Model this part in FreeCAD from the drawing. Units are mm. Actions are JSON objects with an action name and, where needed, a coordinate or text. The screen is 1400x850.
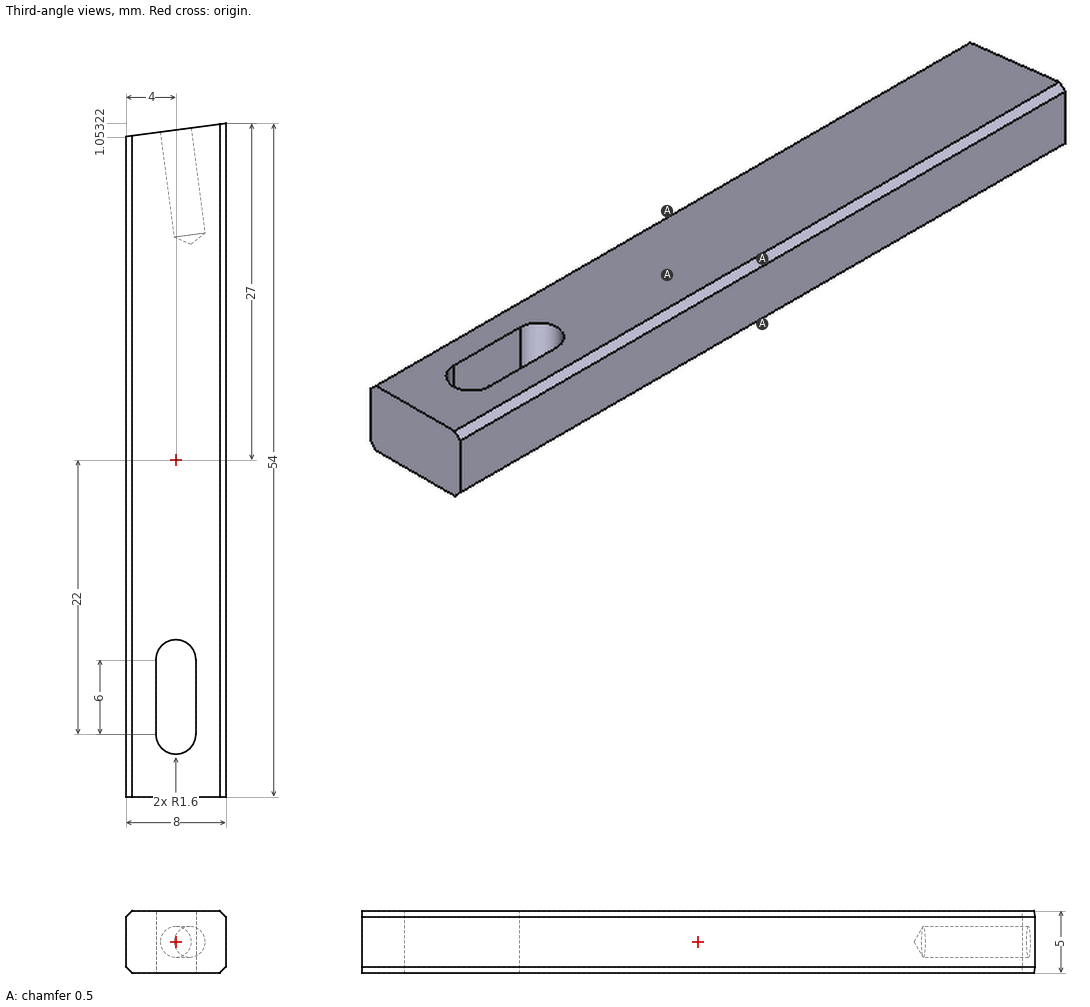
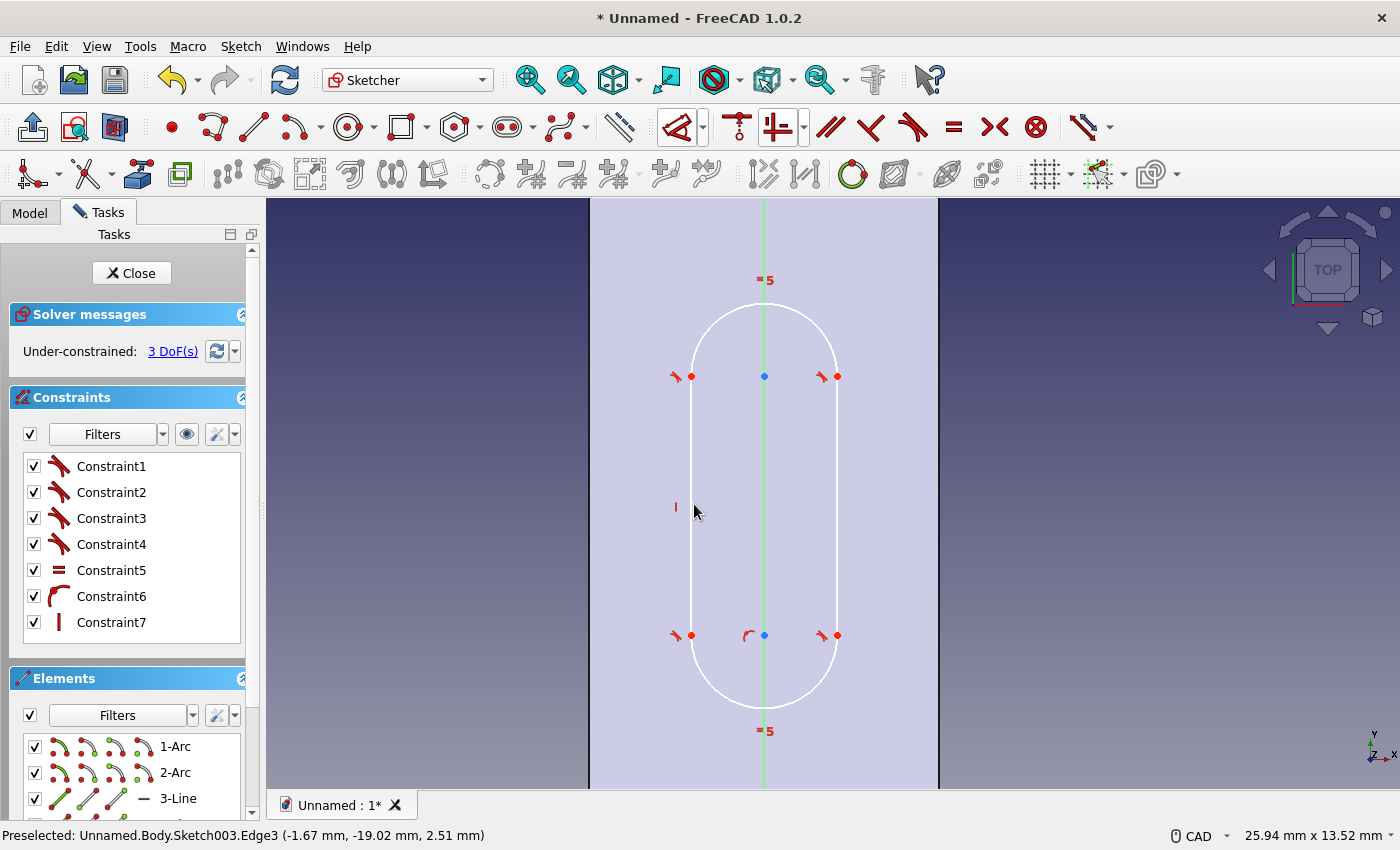
{"action": "left_click", "coordinate": [721, 694]}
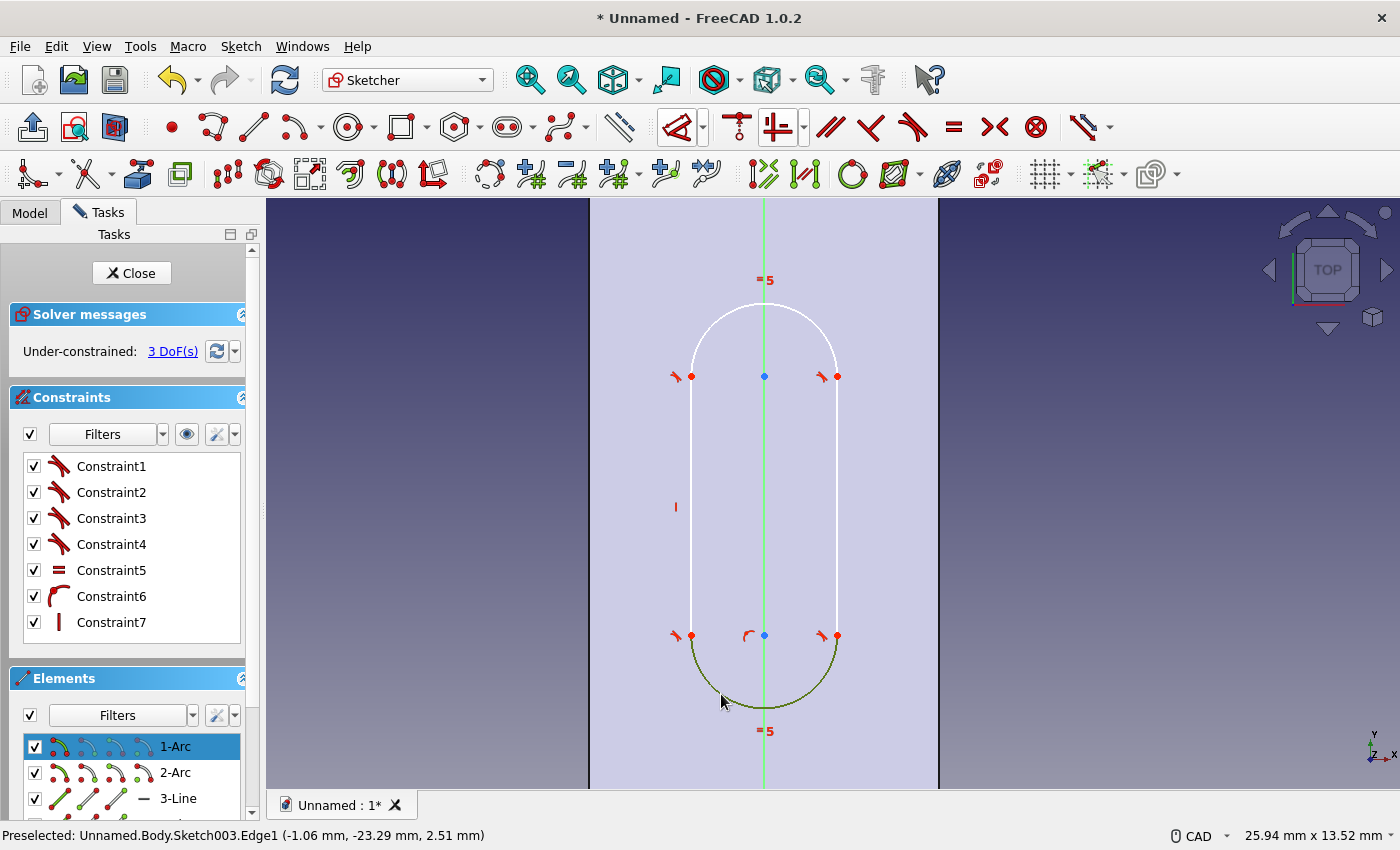
{"action": "key", "text": "k r"}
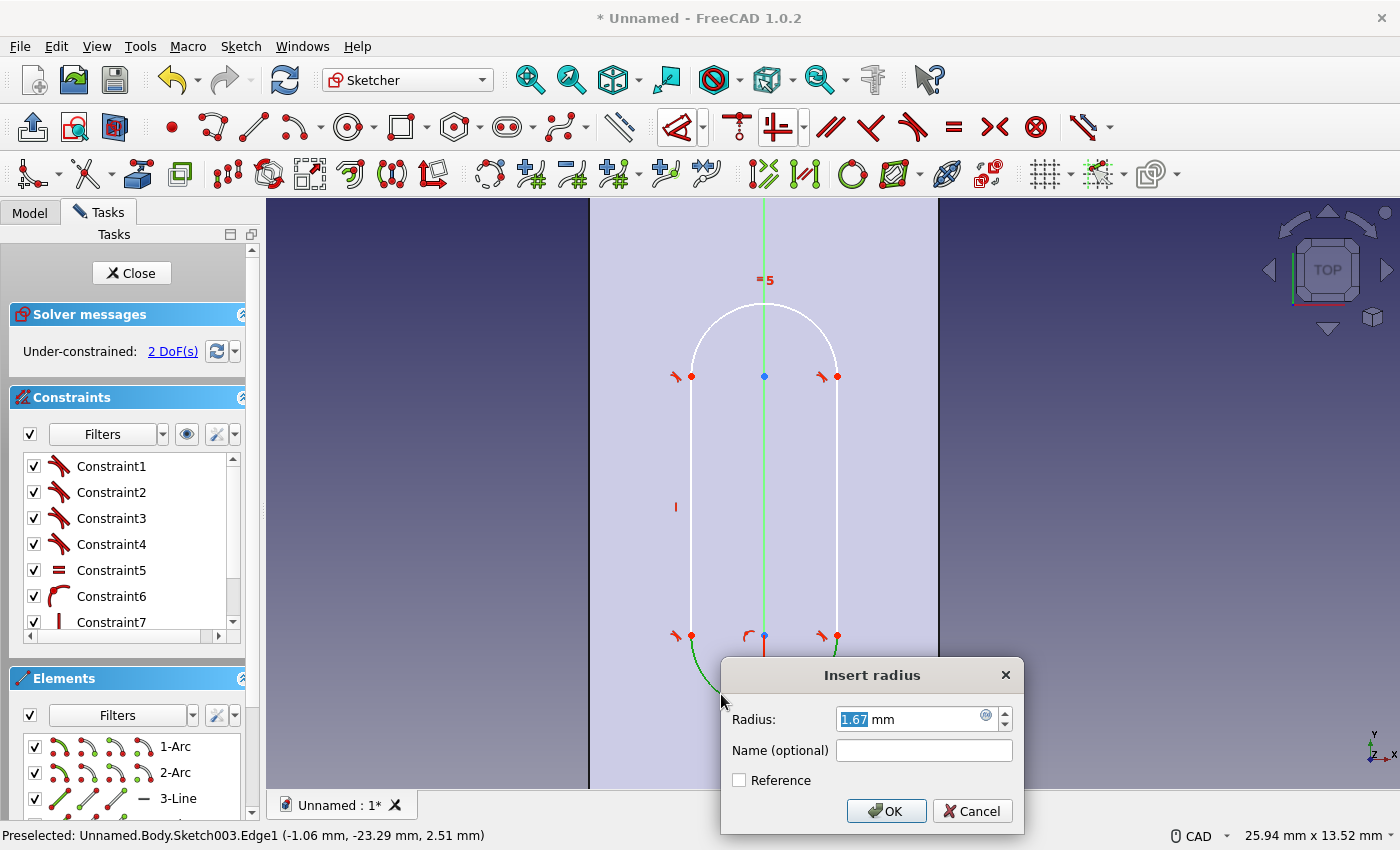
{"action": "type", "text": "1.6"}
{"action": "key", "text": "Return"}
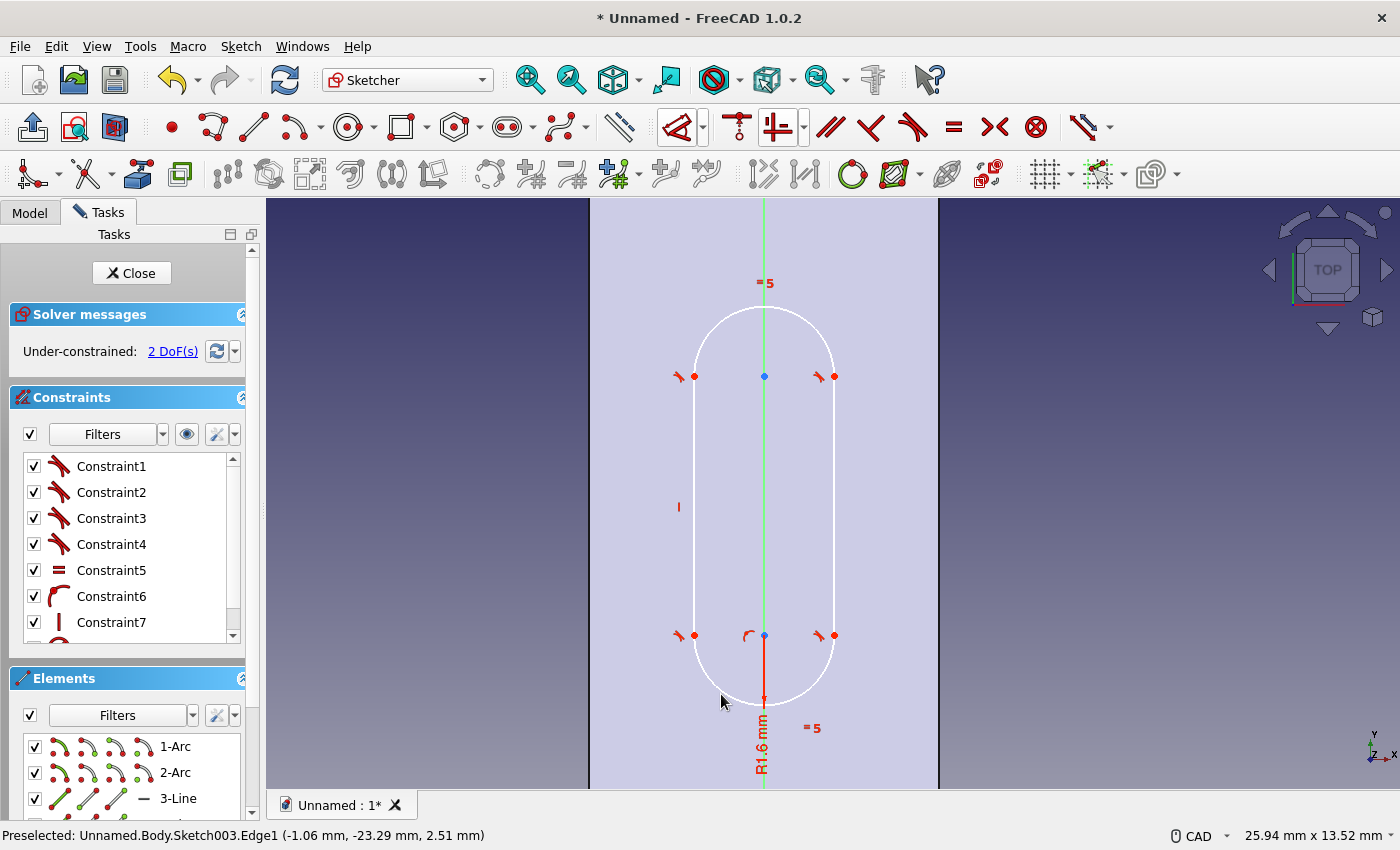
{"action": "left_click", "coordinate": [694, 558]}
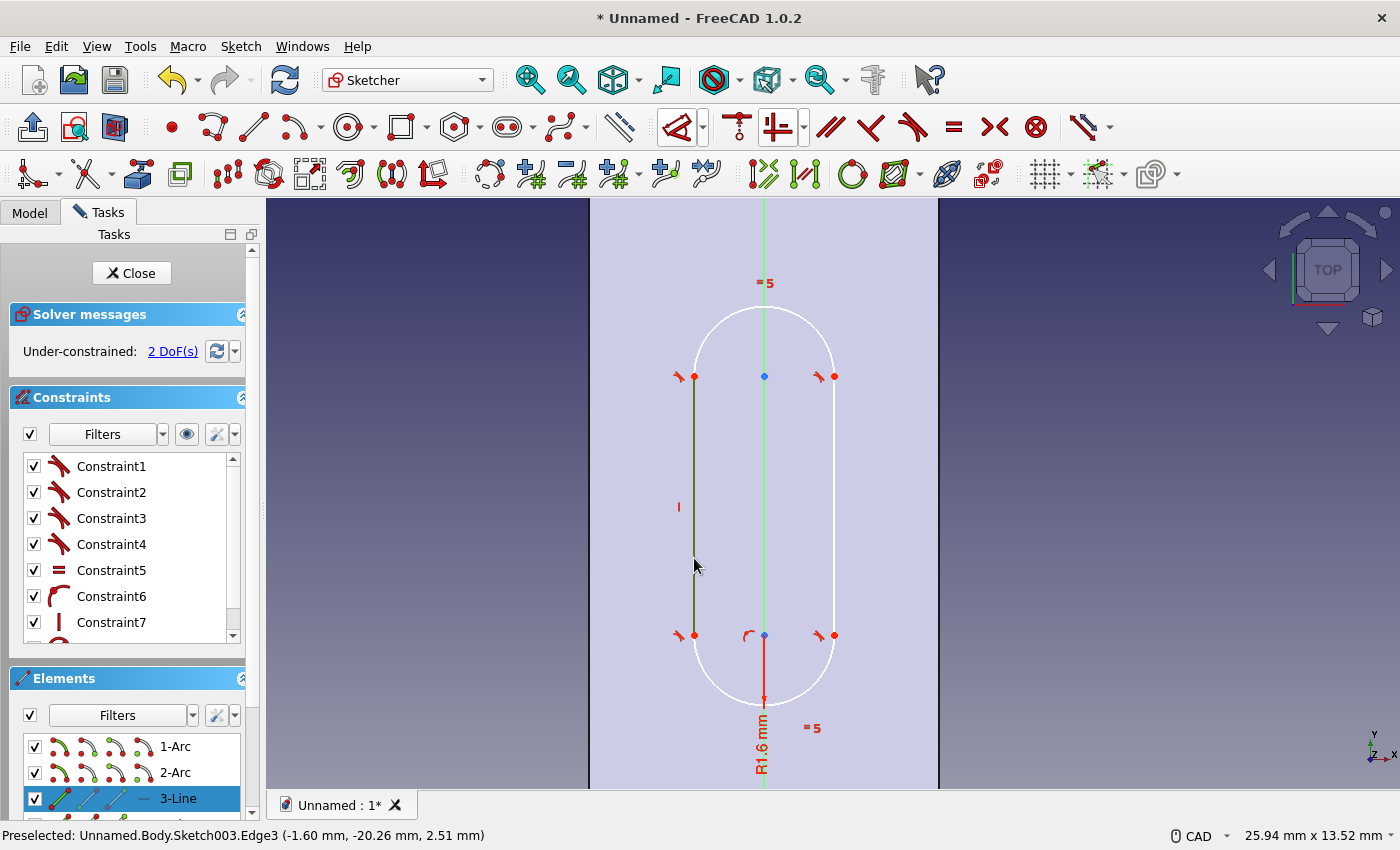
{"action": "key", "text": "i"}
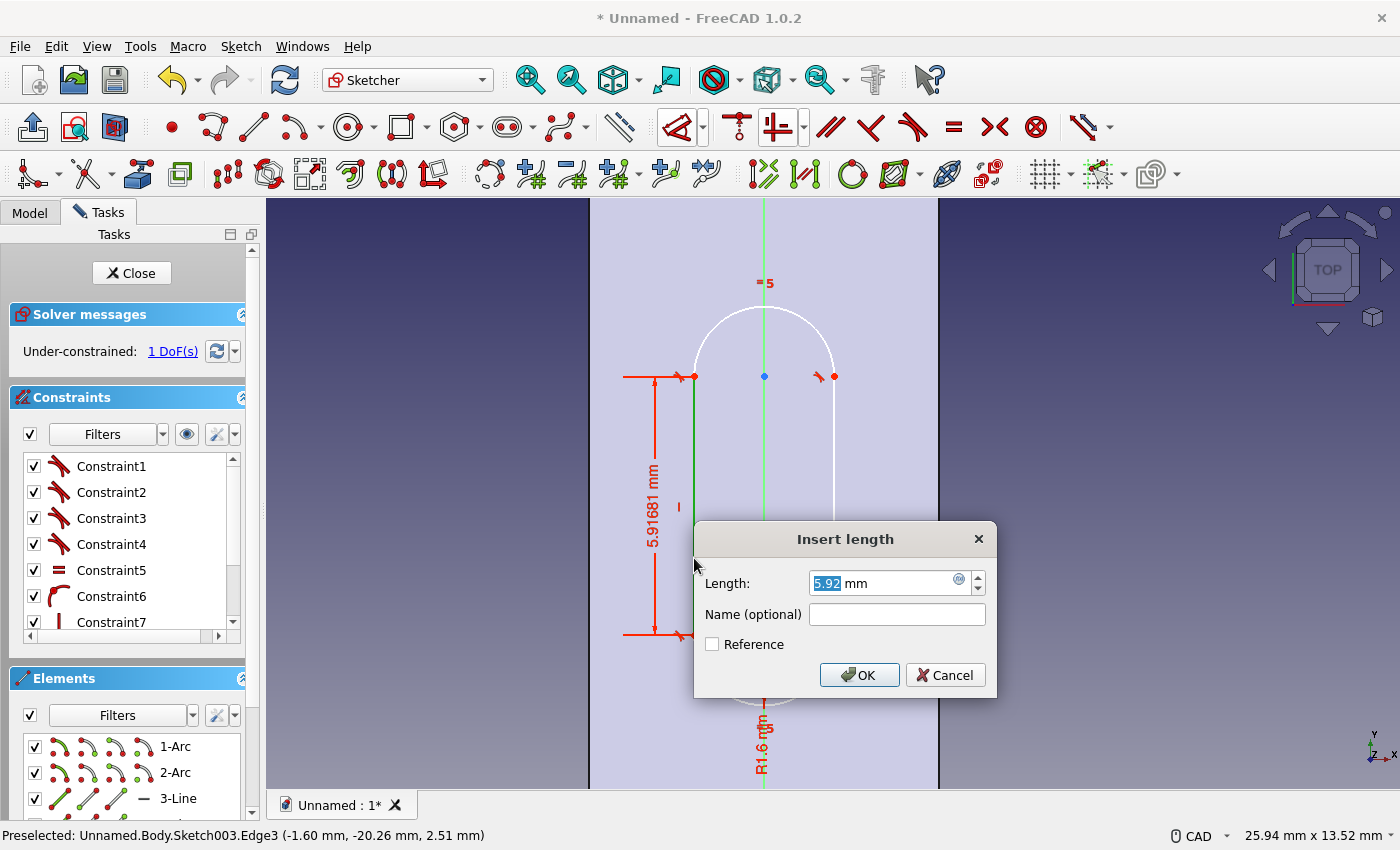
{"action": "type", "text": "6"}
{"action": "key", "text": "Return"}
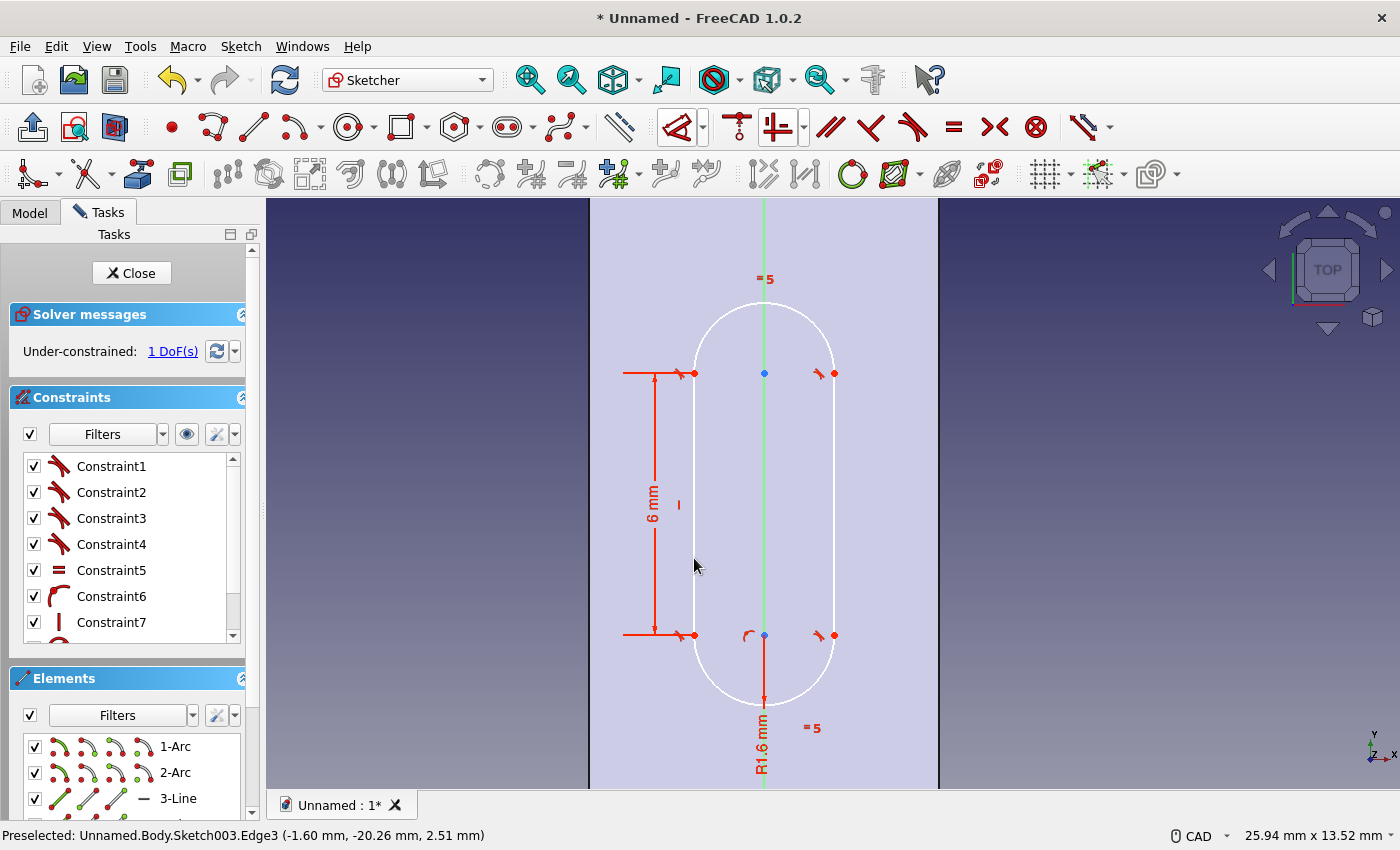
{"action": "left_click", "coordinate": [694, 635]}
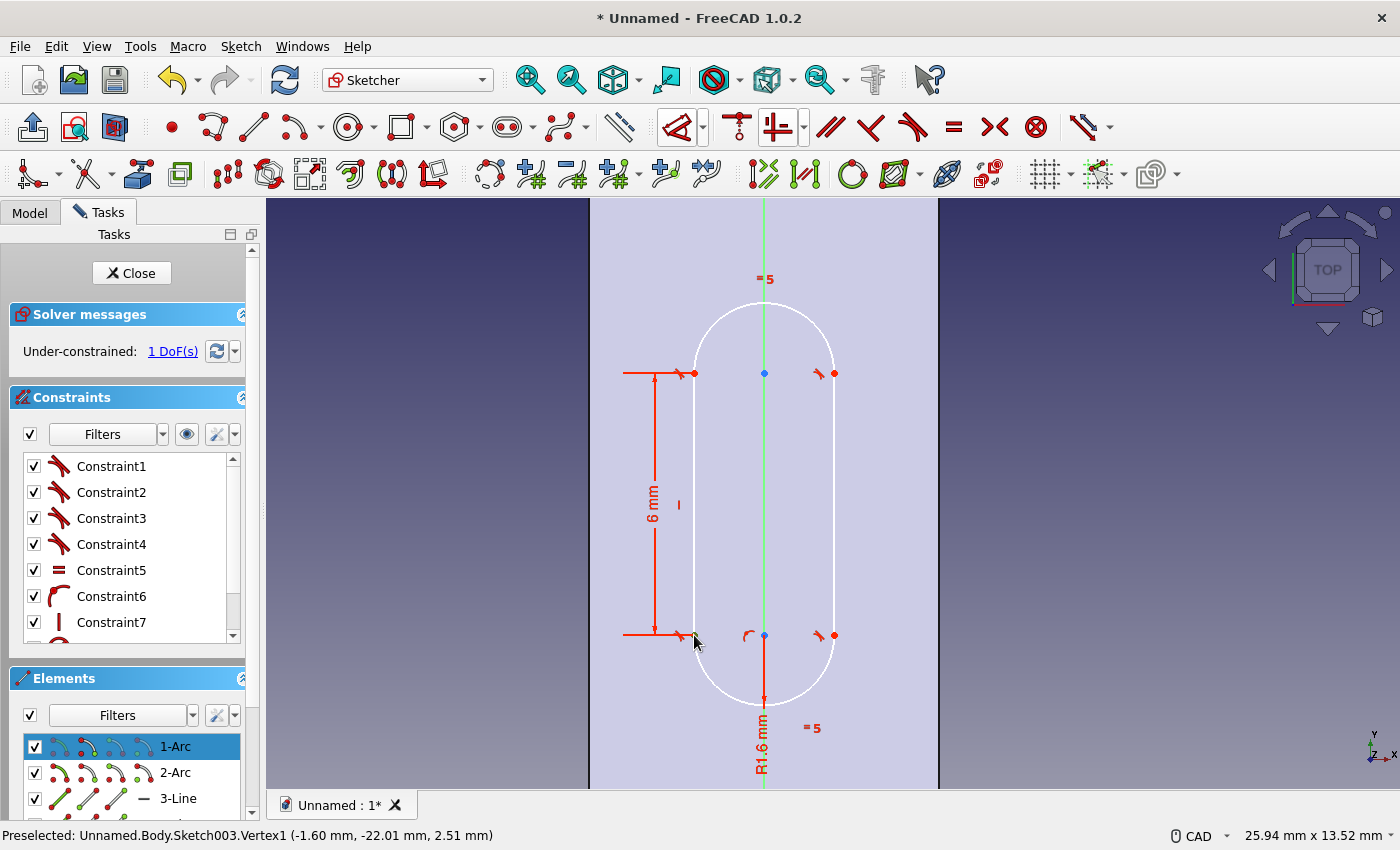
{"action": "left_click", "coordinate": [702, 128]}